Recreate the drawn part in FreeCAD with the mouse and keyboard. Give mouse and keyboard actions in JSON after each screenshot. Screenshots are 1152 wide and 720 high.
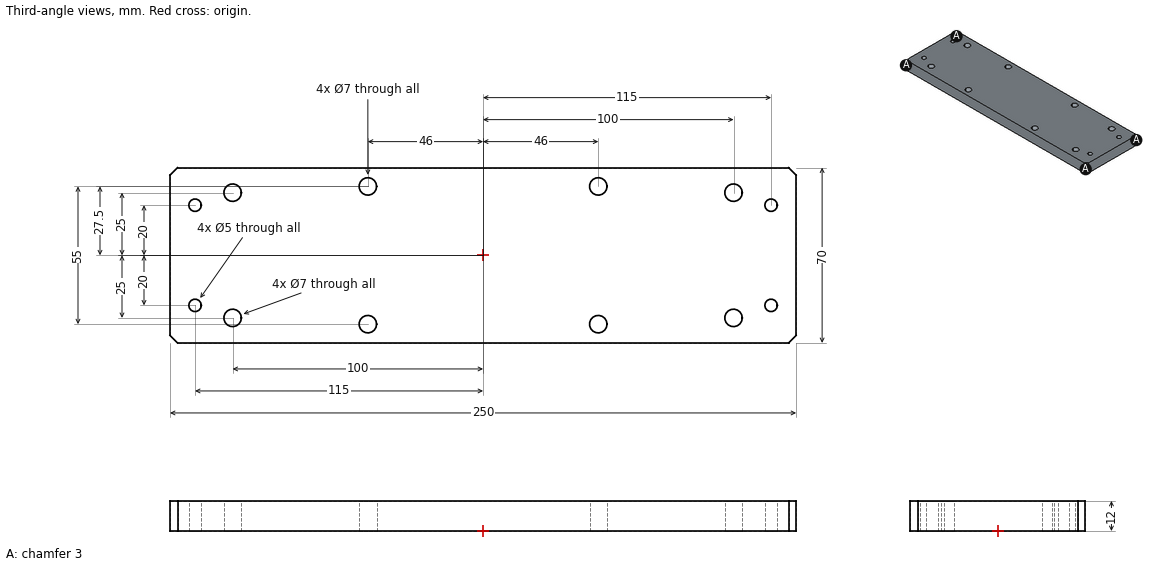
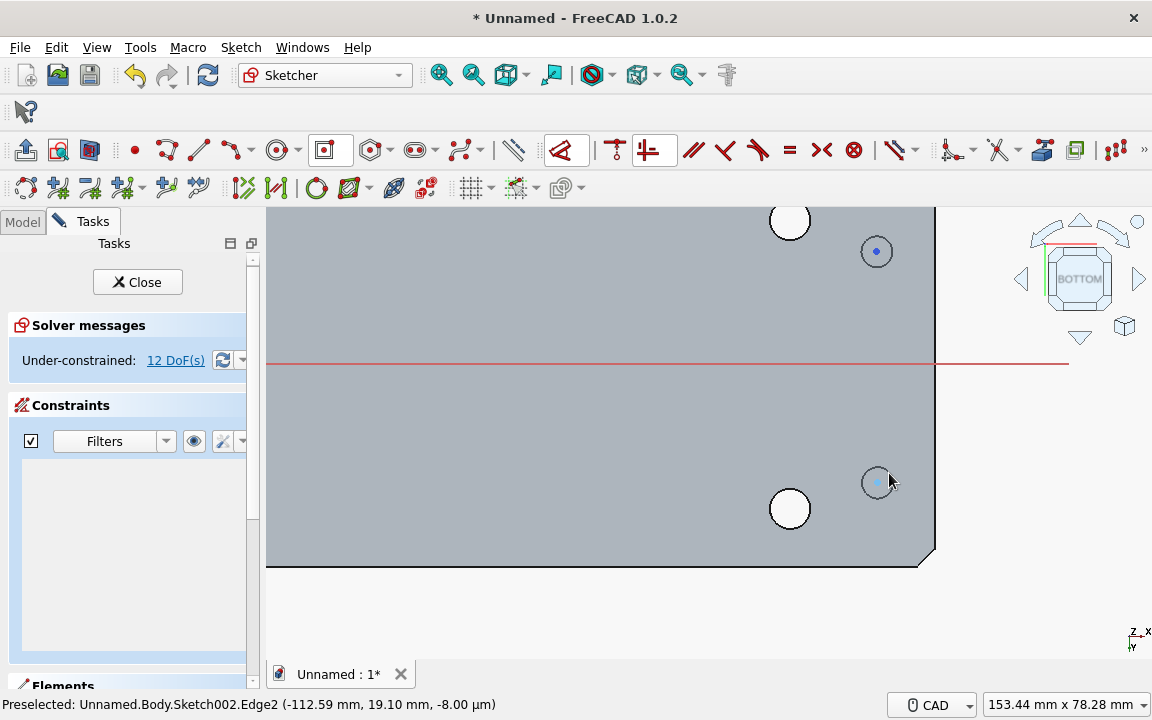
{"action": "left_click", "coordinate": [889, 472]}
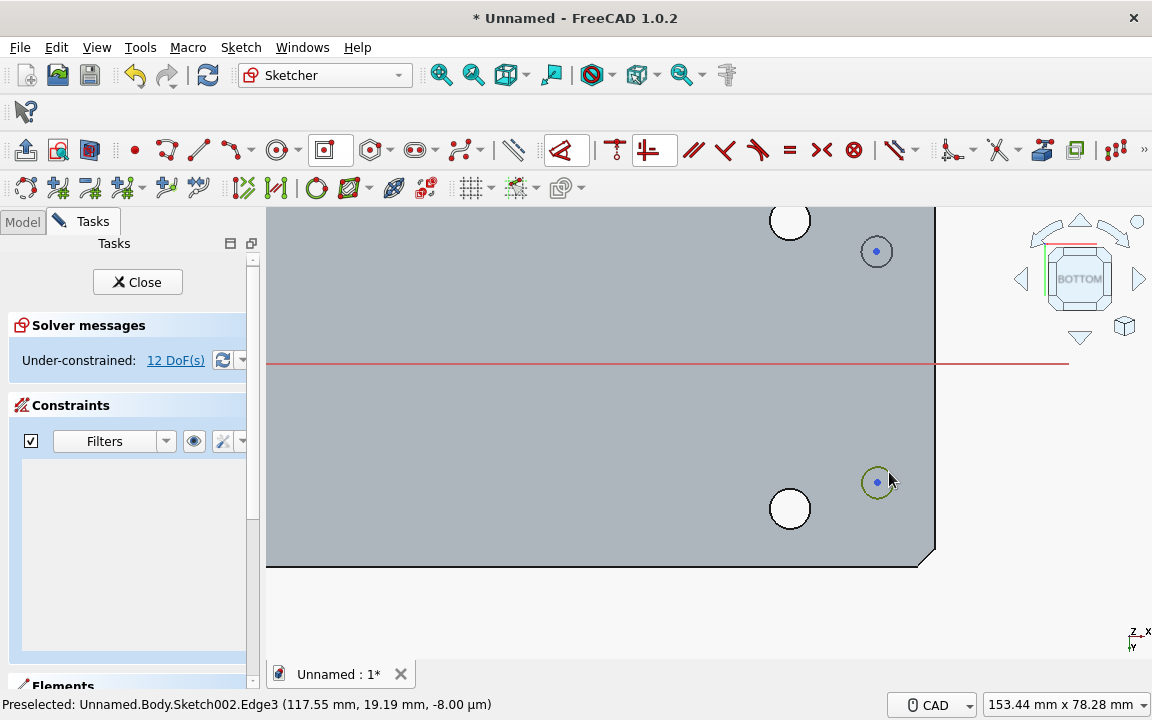
{"action": "left_click", "coordinate": [888, 241]}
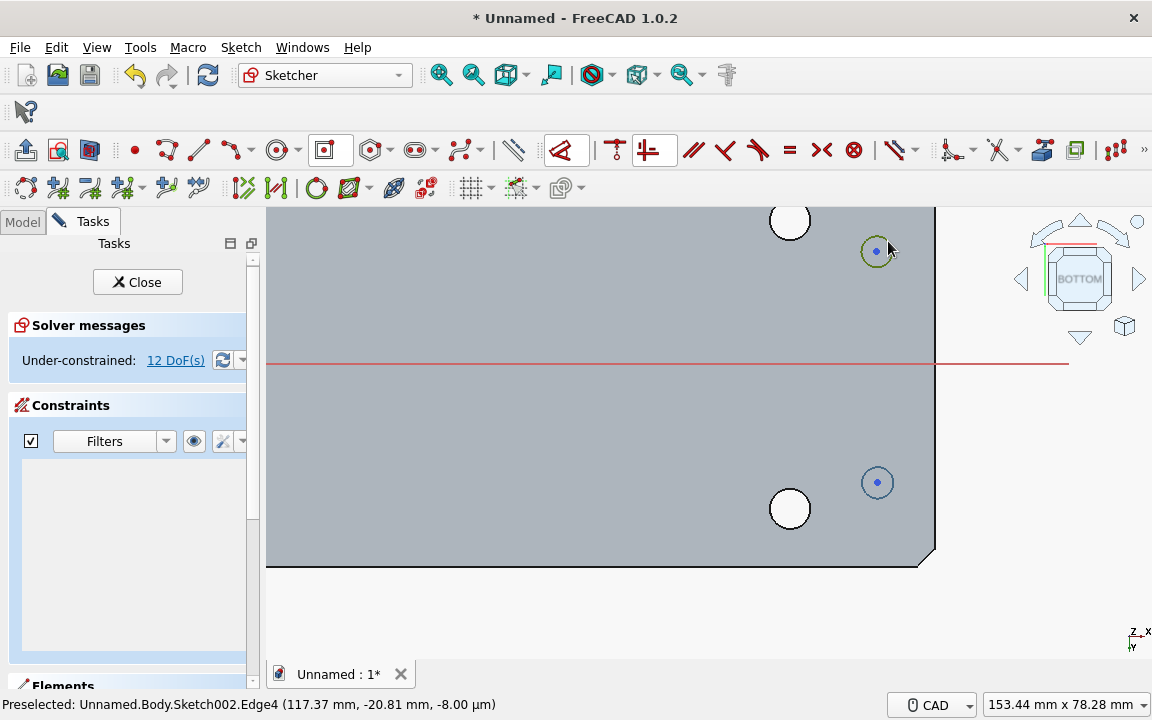
{"action": "key", "text": "e"}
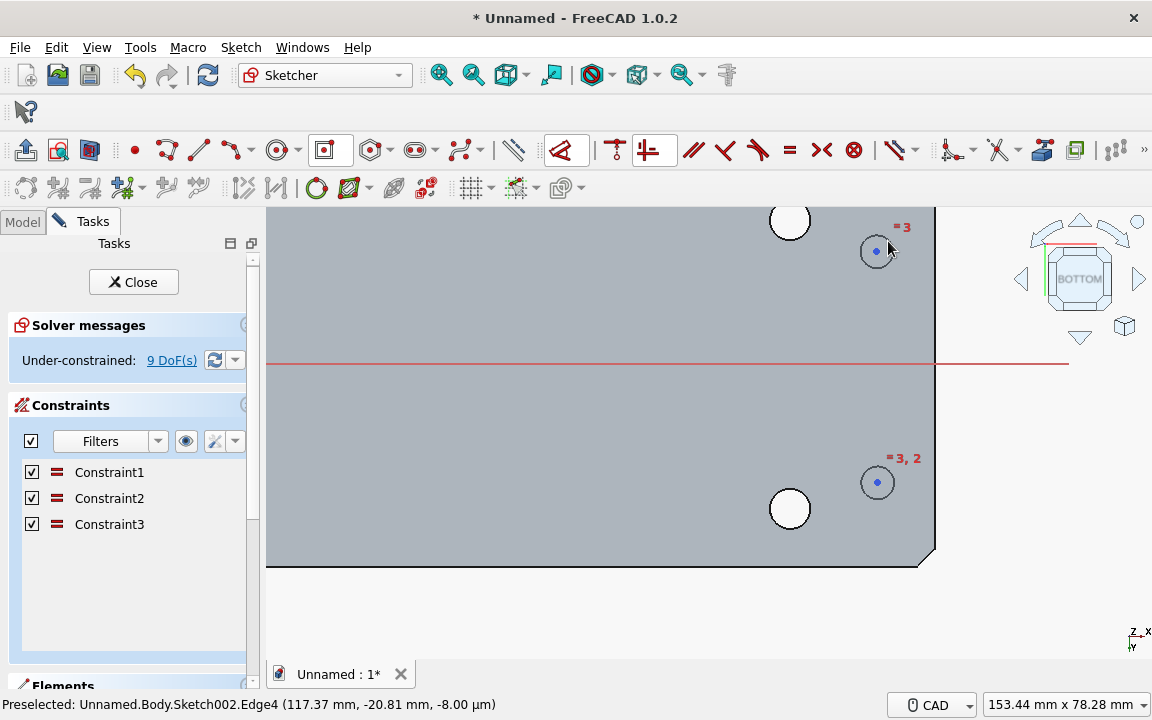
{"action": "scroll", "coordinate": [889, 473], "scroll_direction": "down", "scroll_amount": 5}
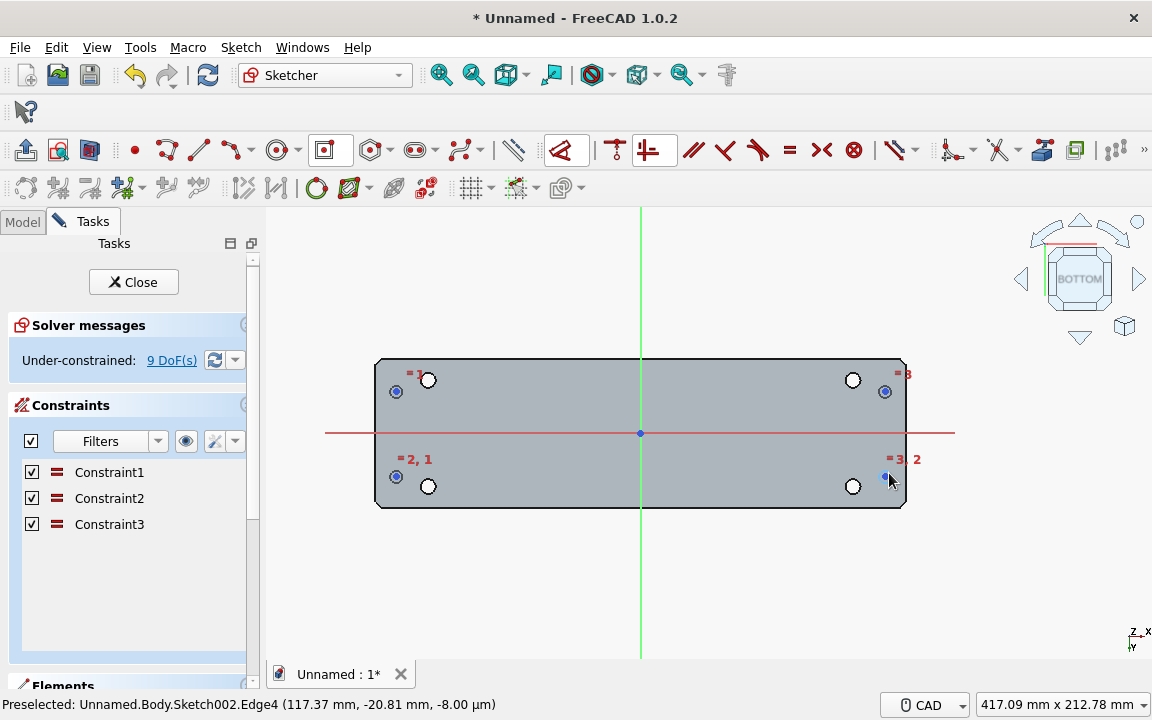
{"action": "left_click", "coordinate": [396, 392]}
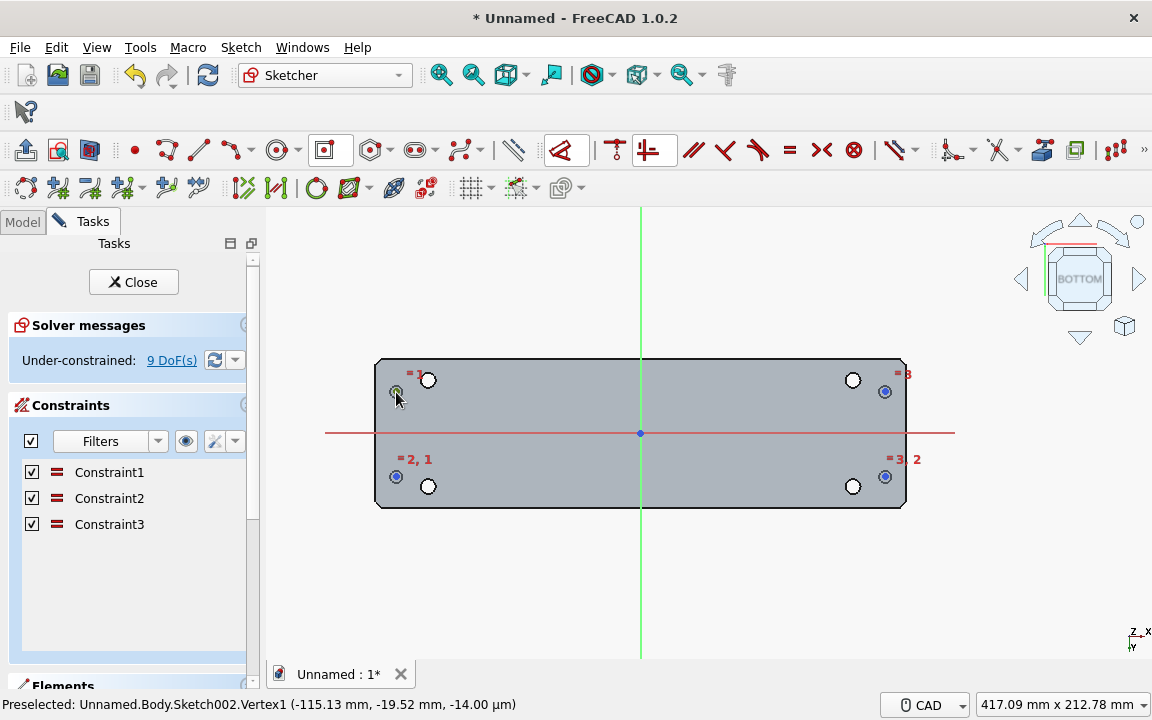
{"action": "left_click", "coordinate": [396, 477]}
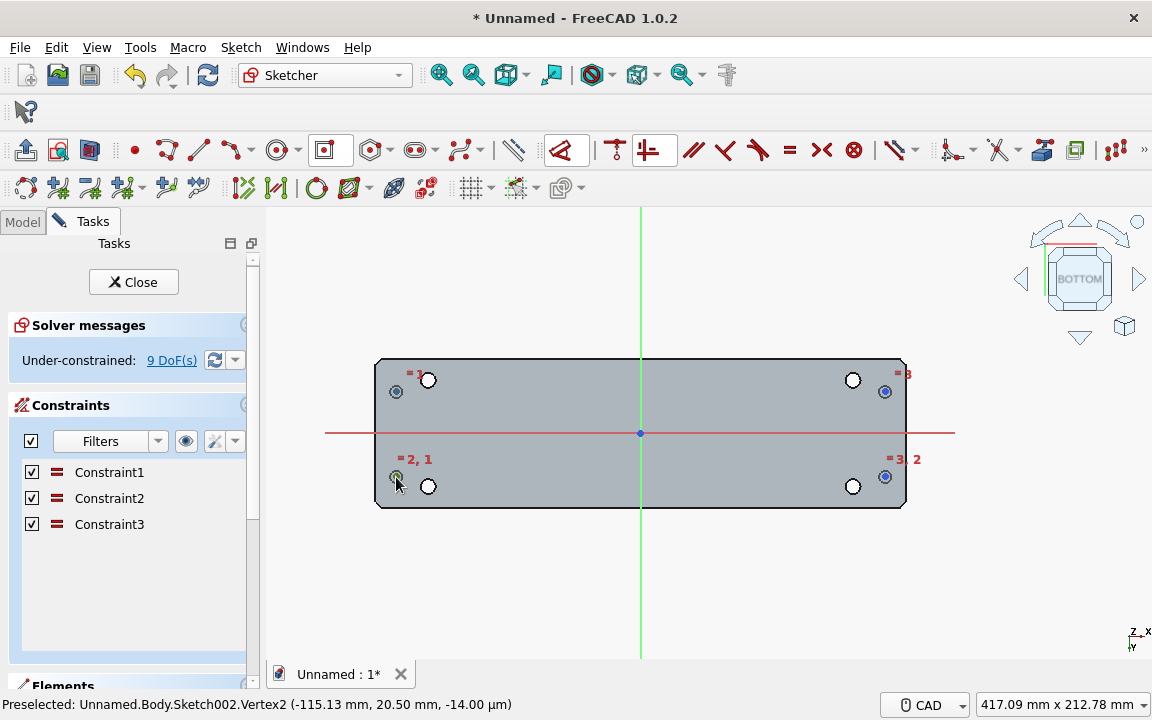
{"action": "left_click", "coordinate": [672, 150]}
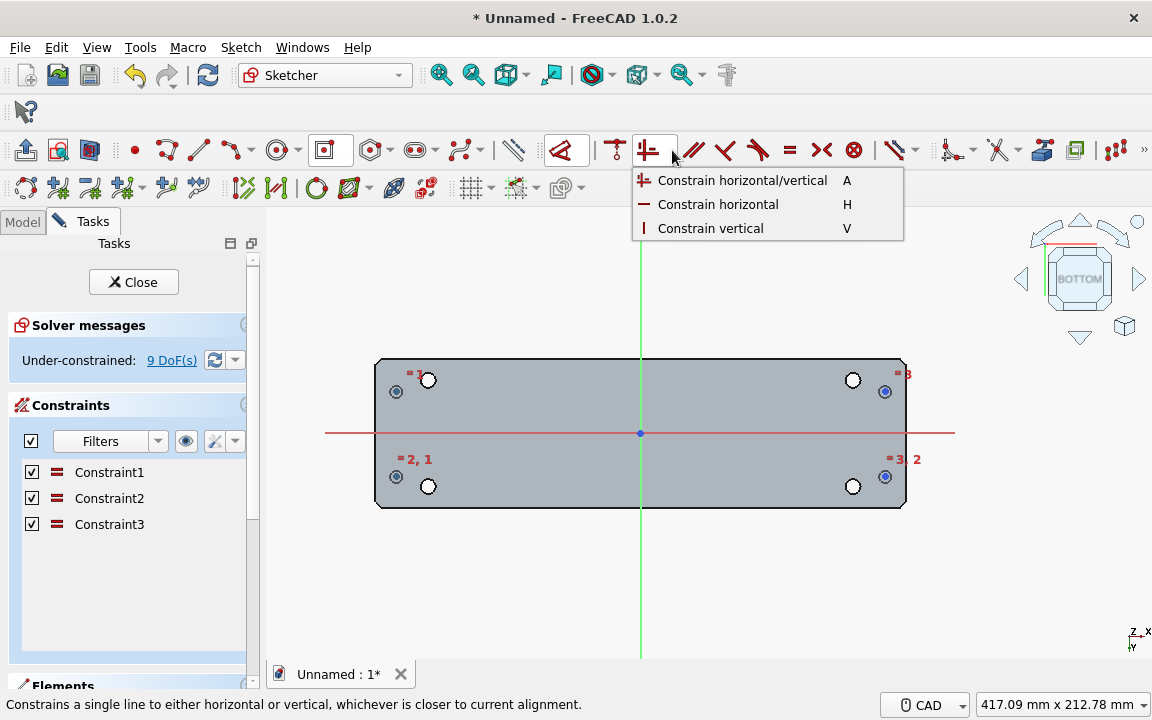
{"action": "left_click", "coordinate": [768, 228]}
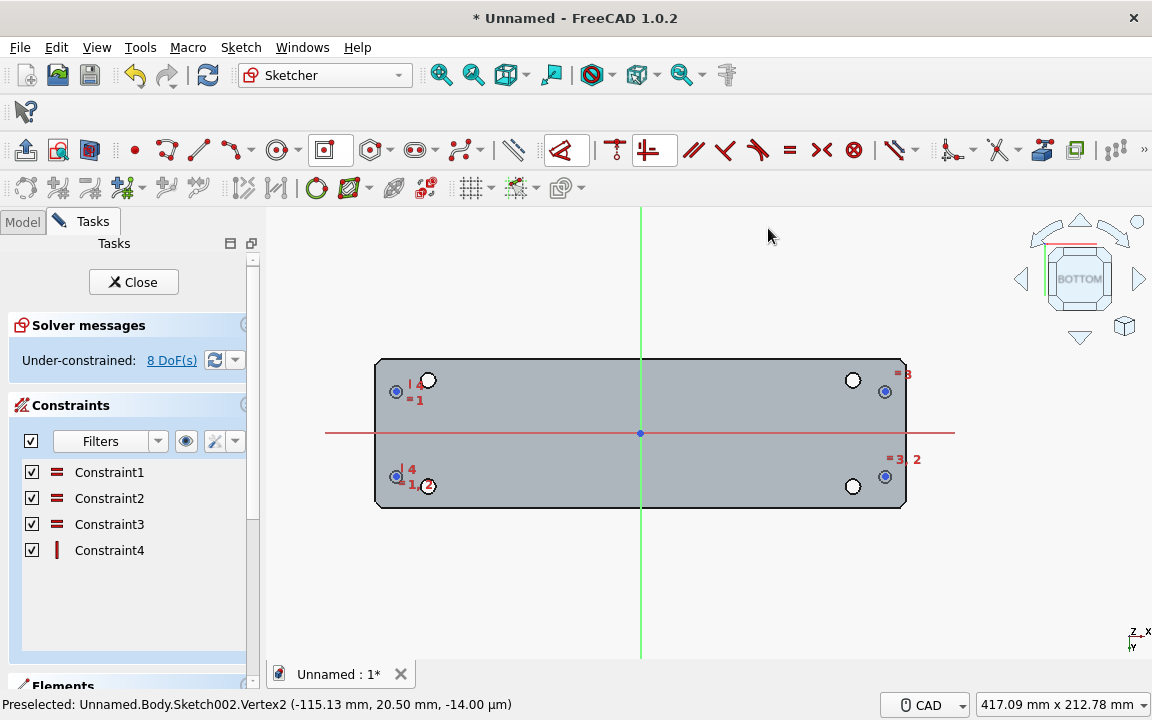
{"action": "left_click", "coordinate": [396, 477]}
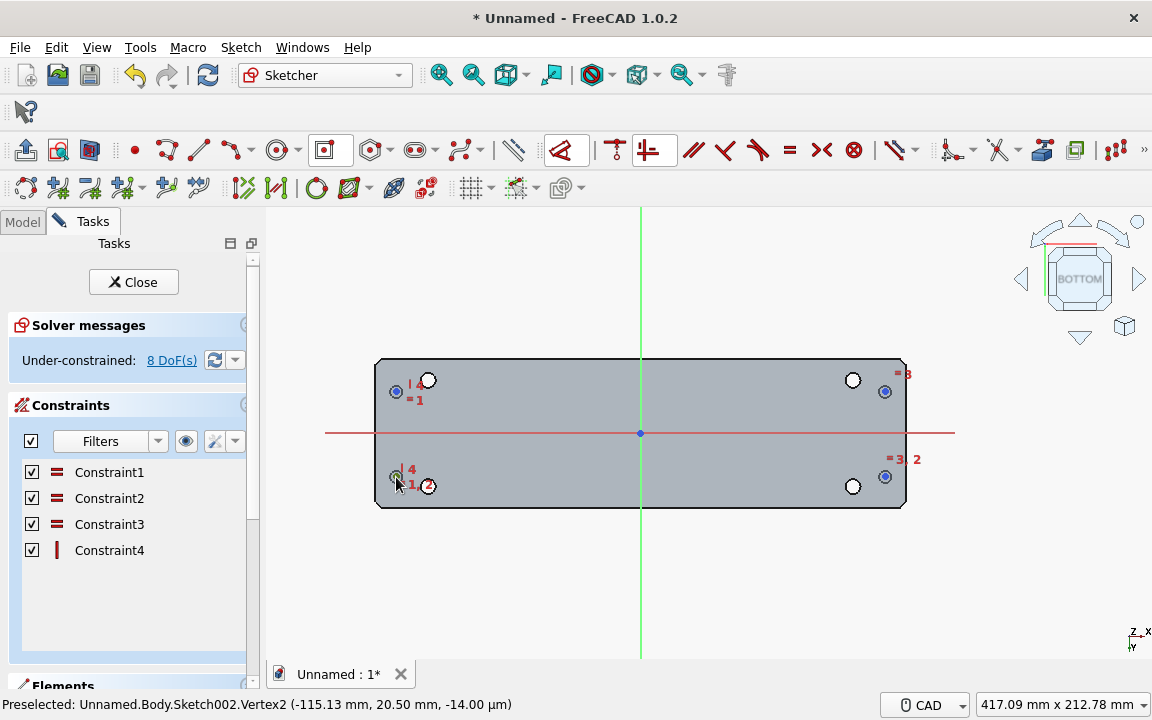
{"action": "left_click", "coordinate": [885, 477]}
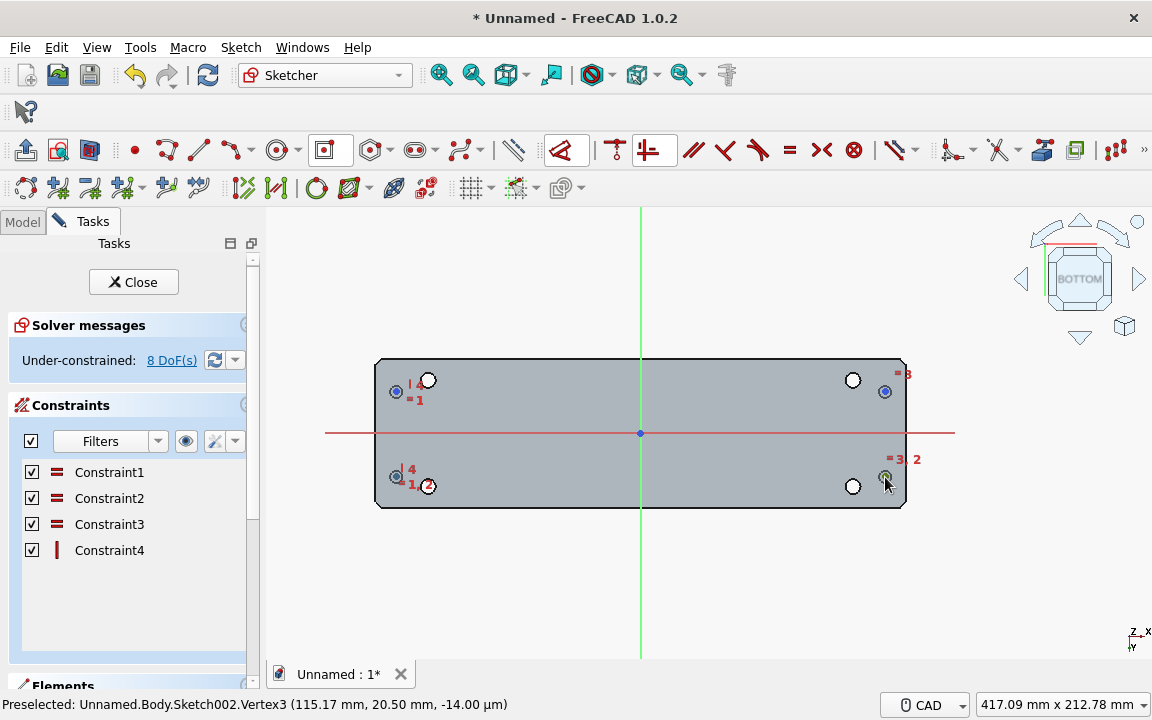
{"action": "key", "text": "h"}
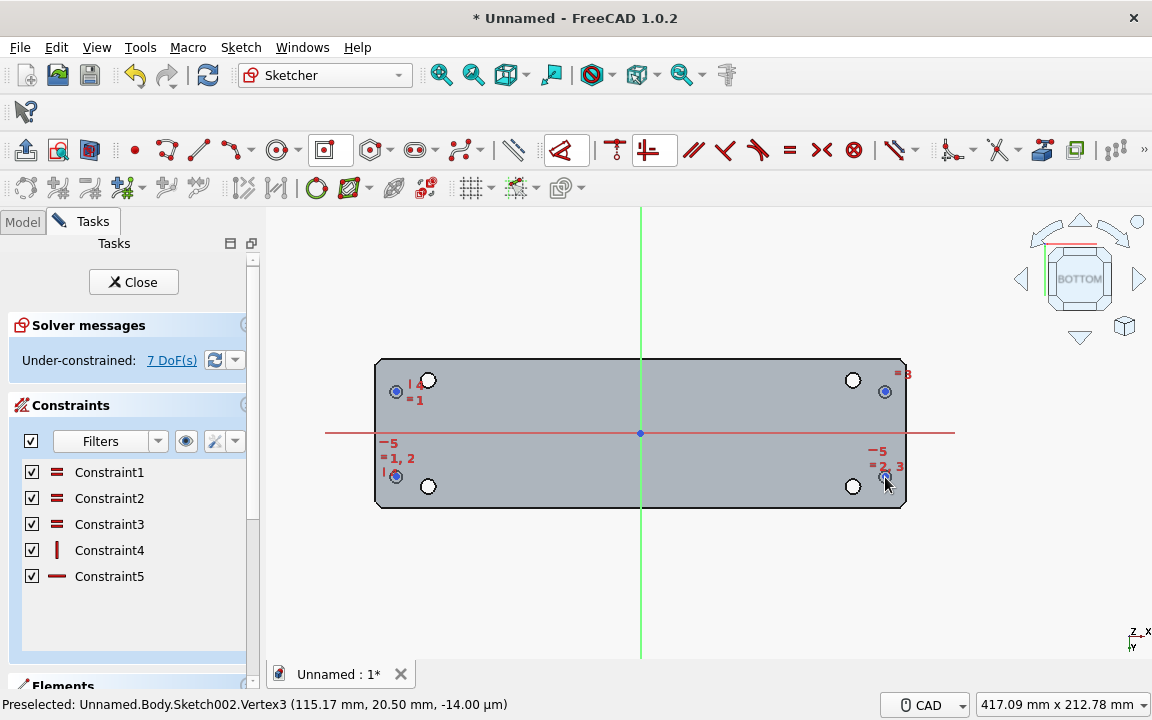
{"action": "left_click", "coordinate": [885, 477]}